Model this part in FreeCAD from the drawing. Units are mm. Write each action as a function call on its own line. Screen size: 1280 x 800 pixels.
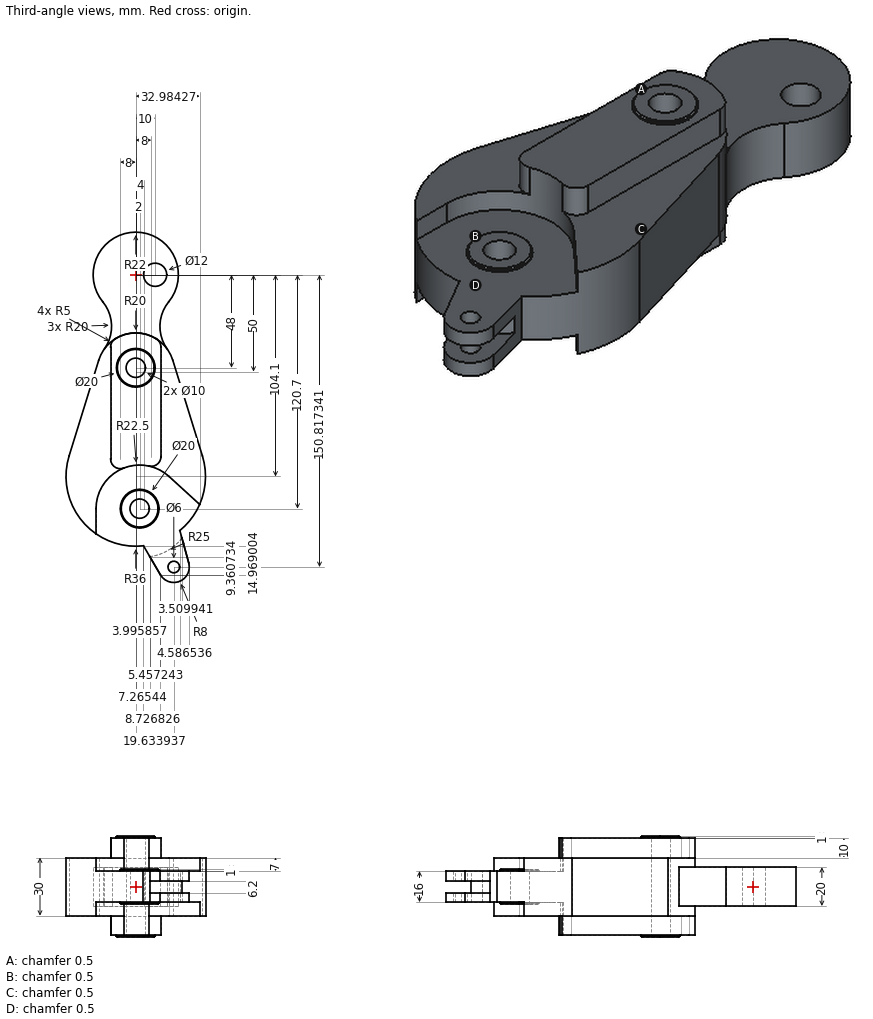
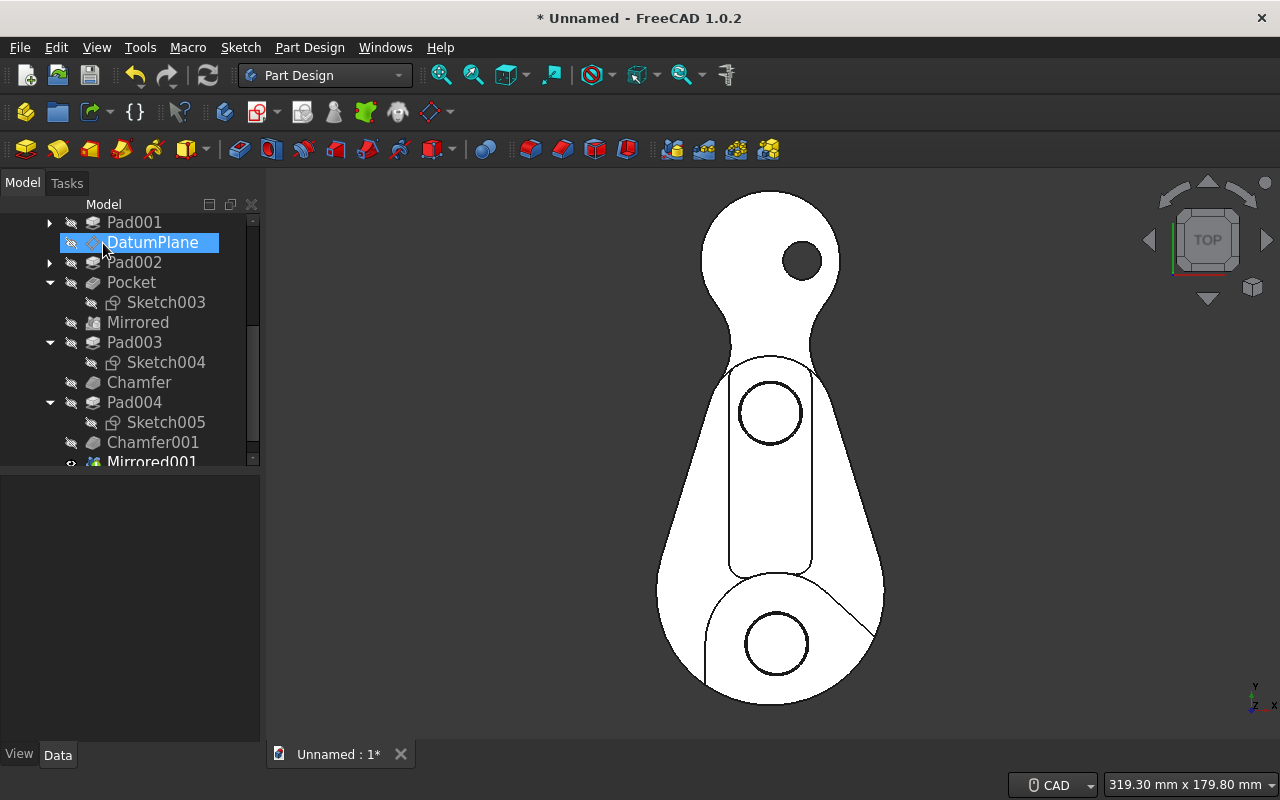
key(1)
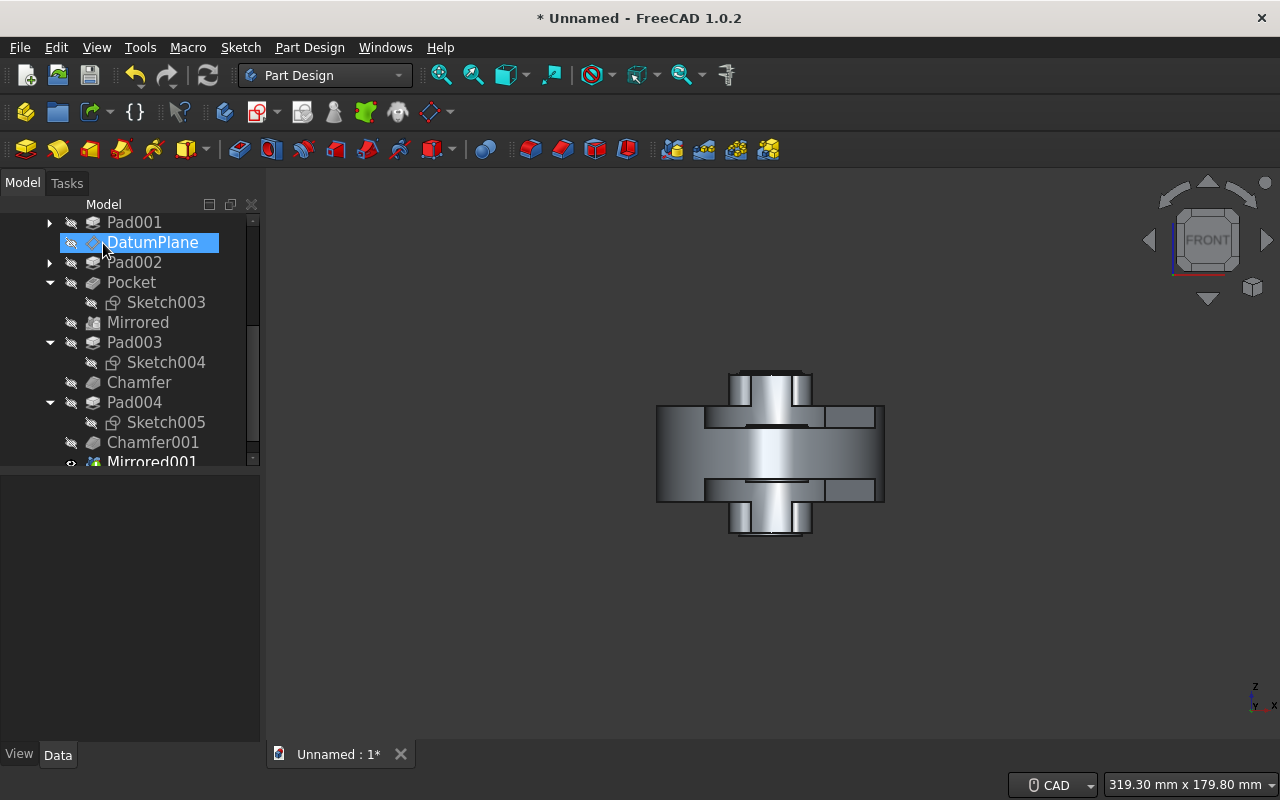
click(442, 76)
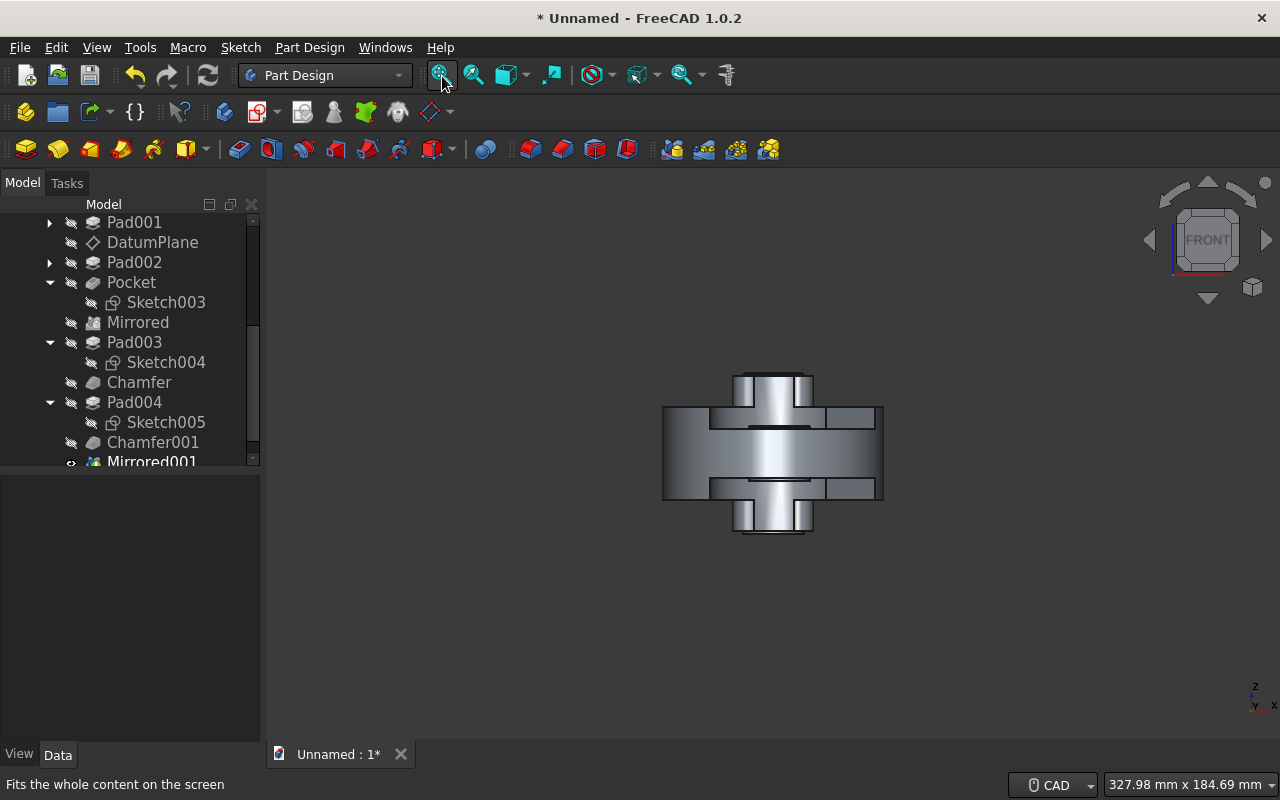
key(3)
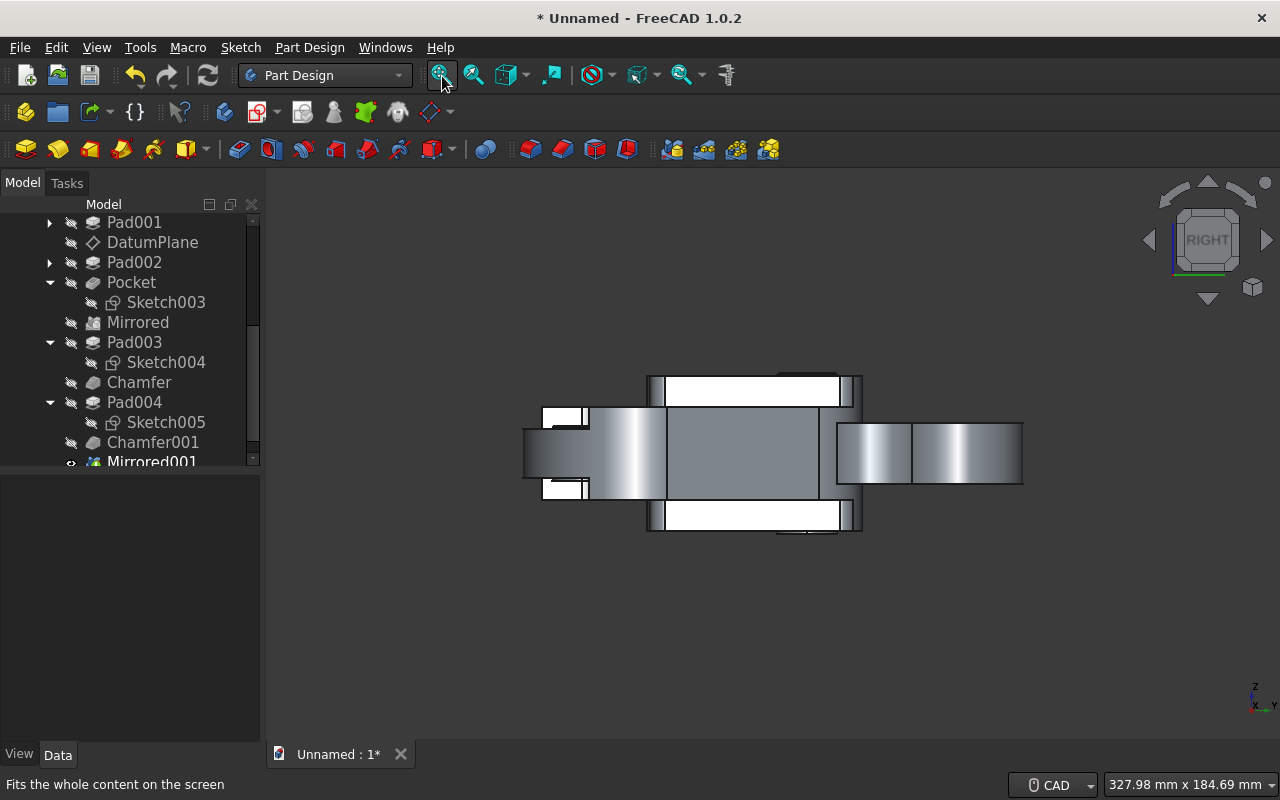
key(5)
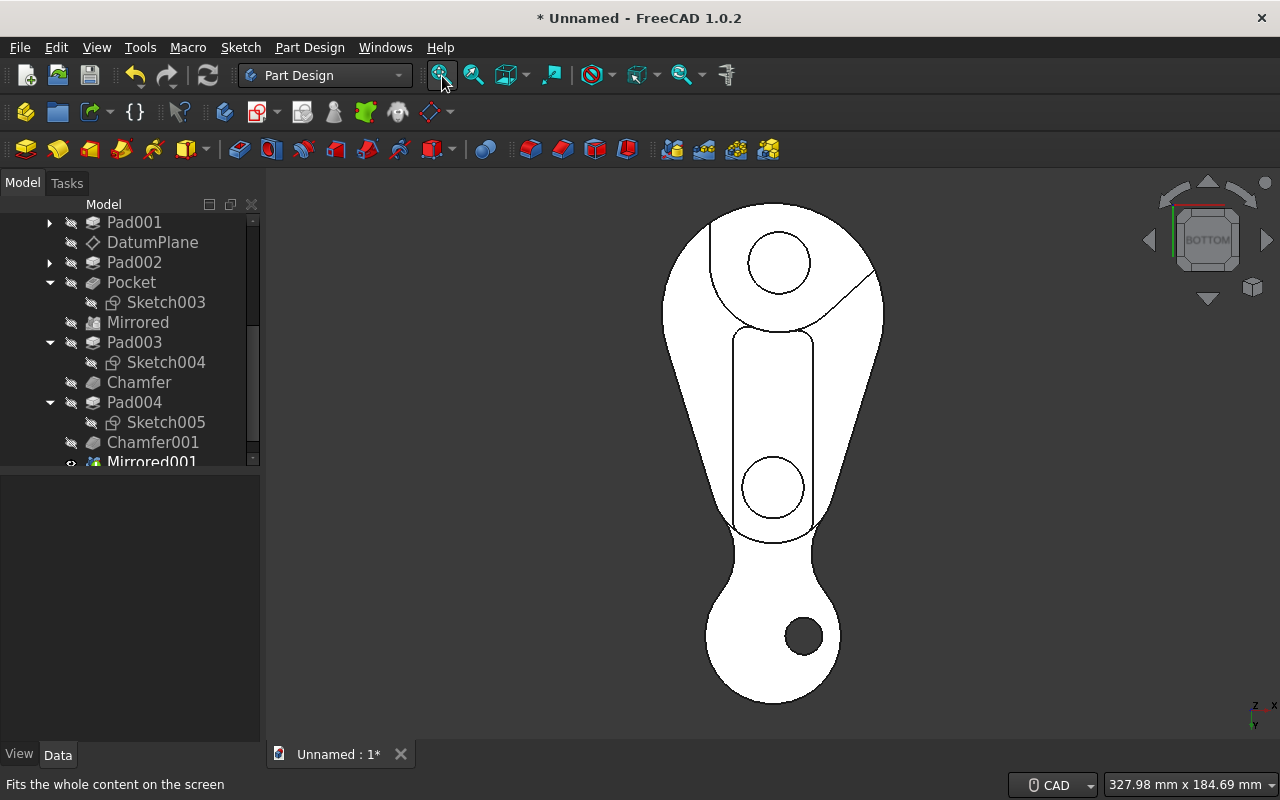
click(742, 487)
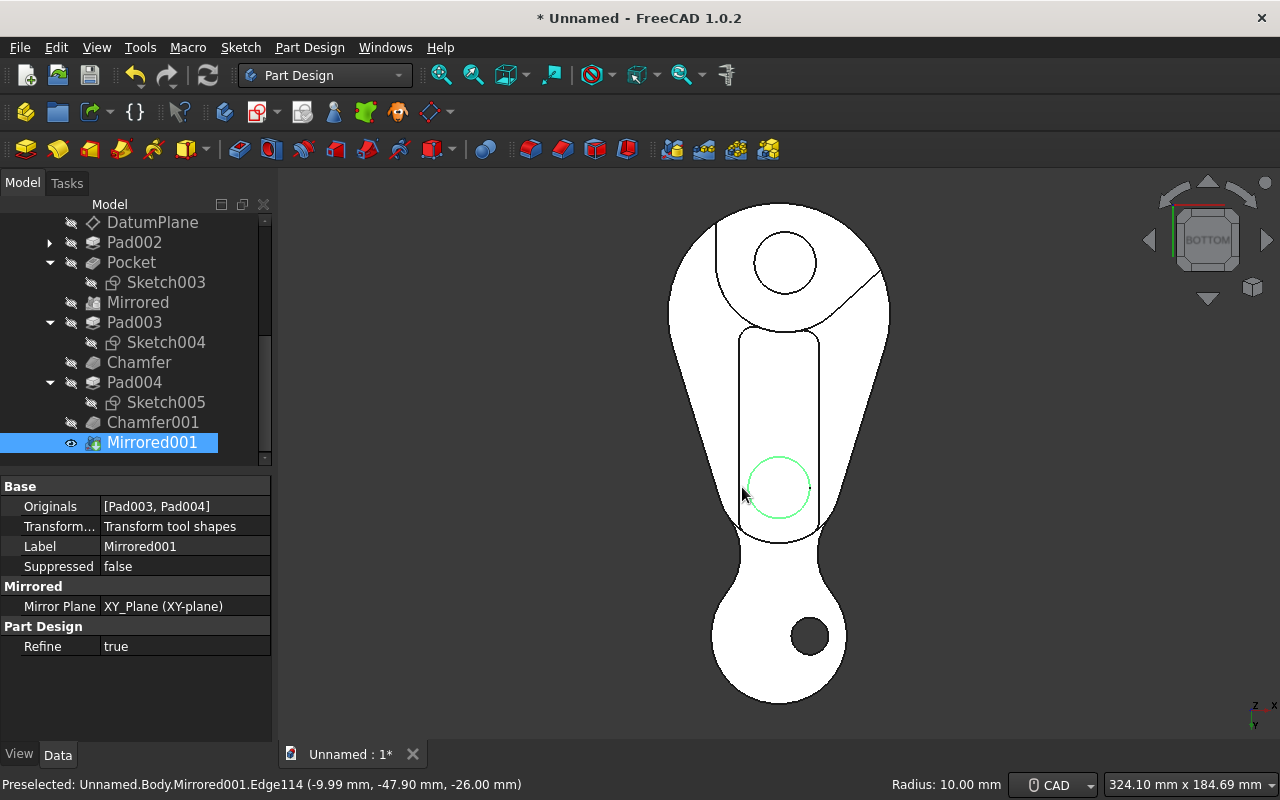
click(564, 150)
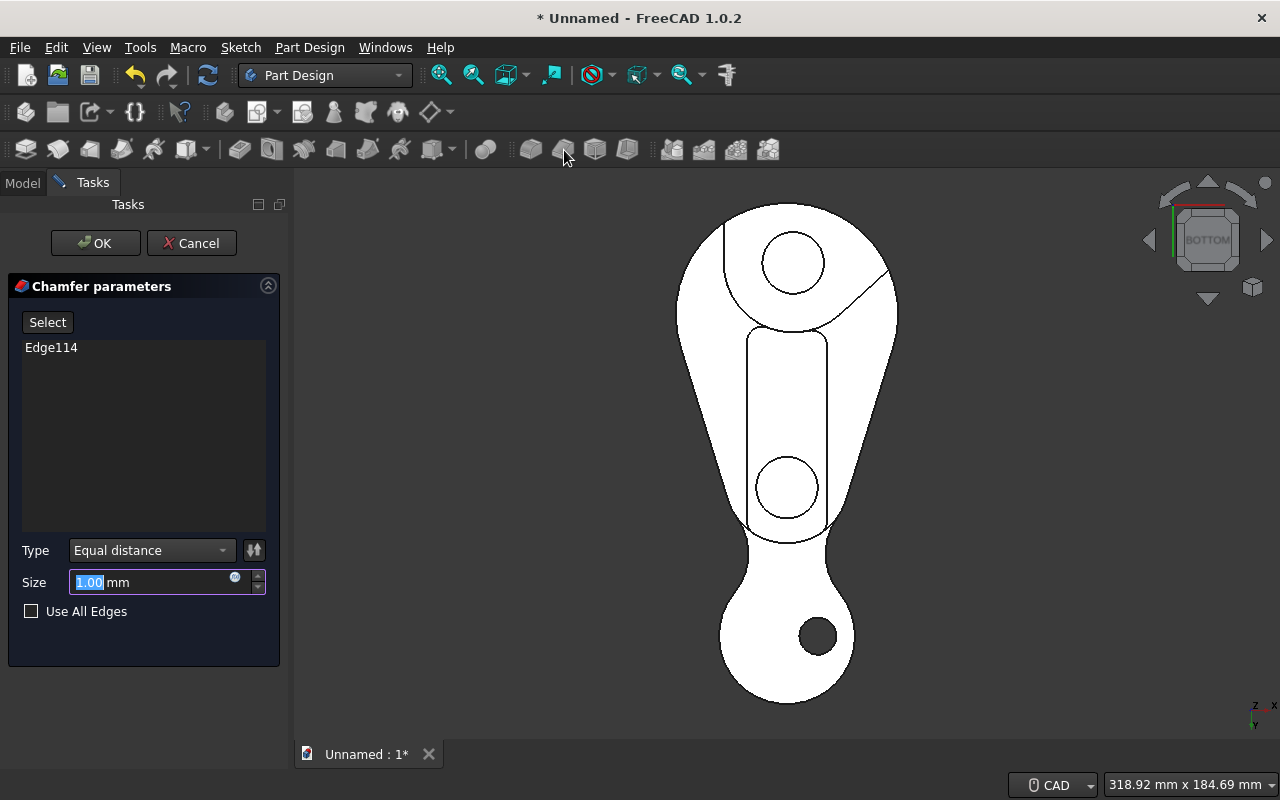
text(0.5)
key(Tab)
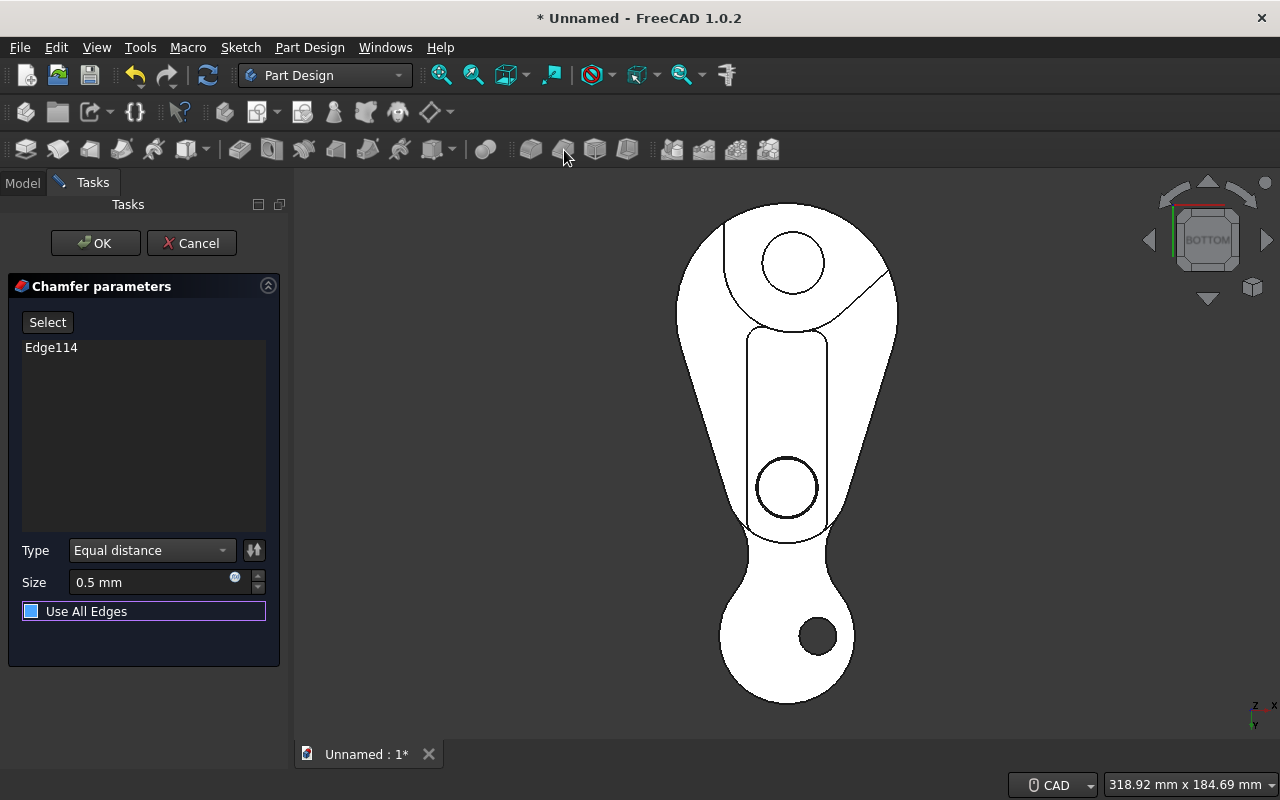
click(96, 243)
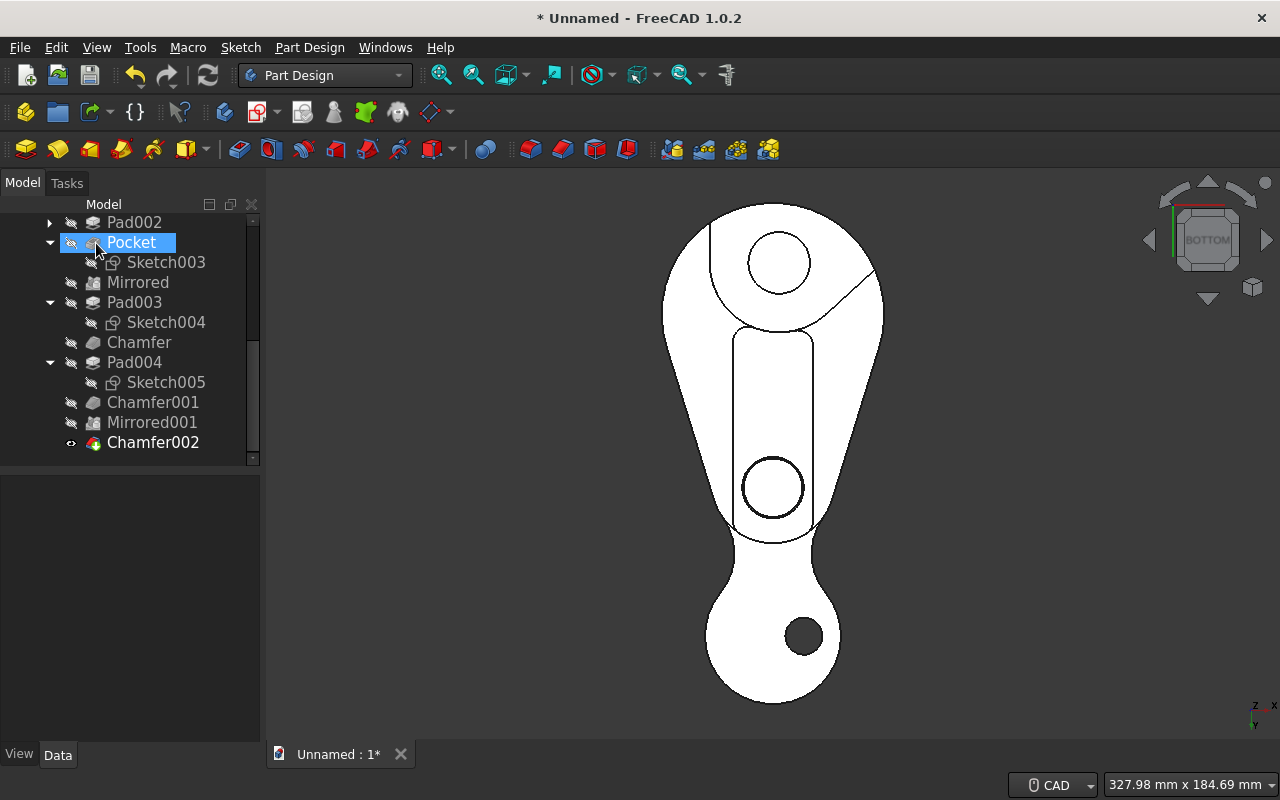
click(748, 262)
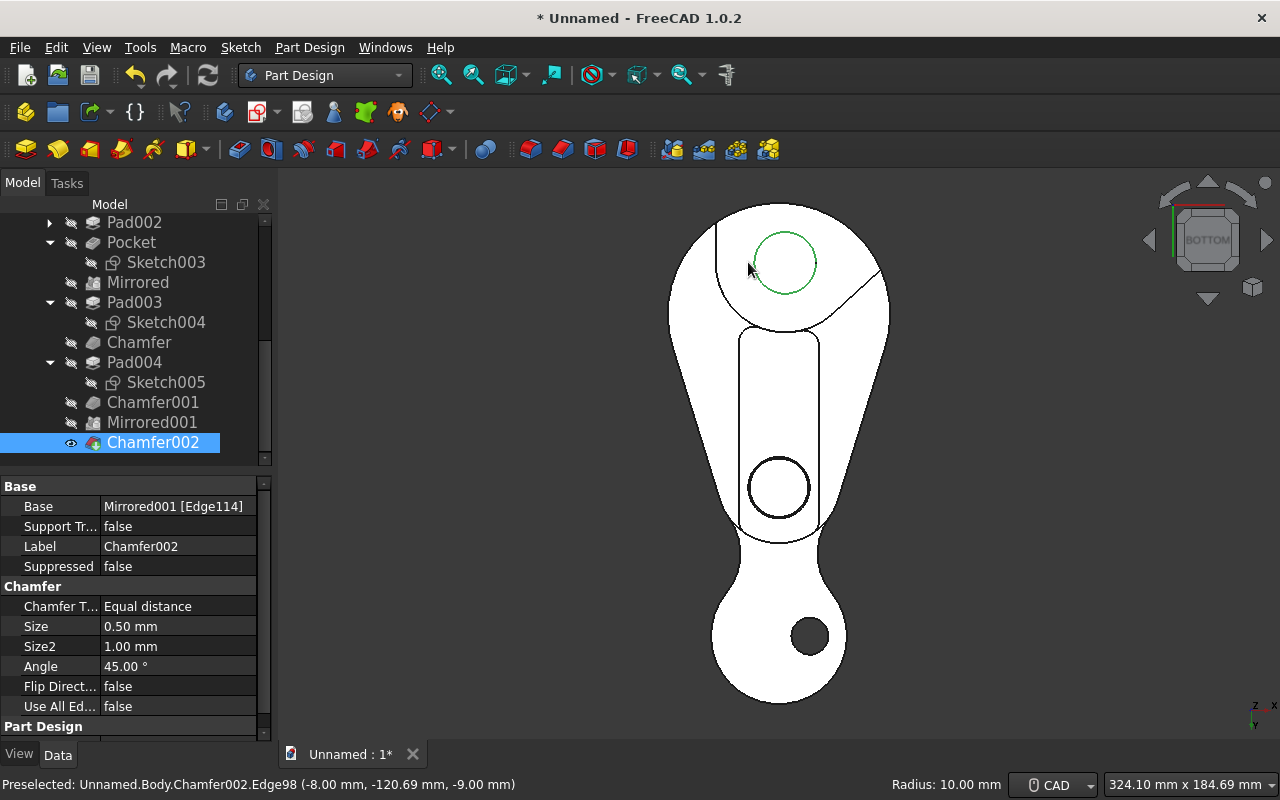
click(564, 150)